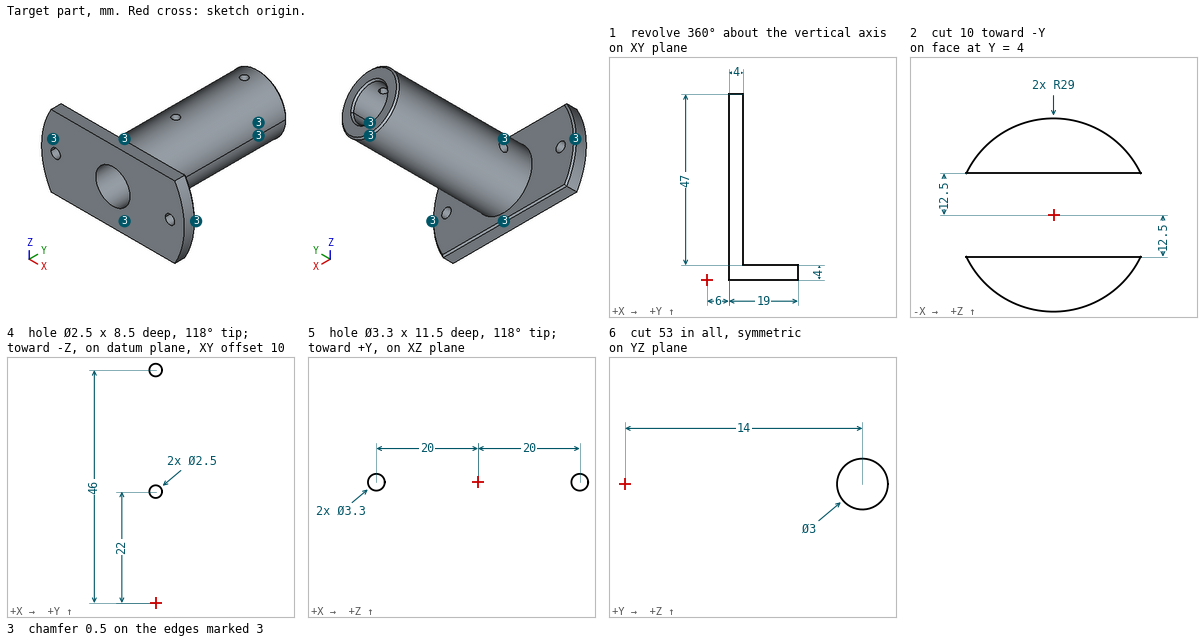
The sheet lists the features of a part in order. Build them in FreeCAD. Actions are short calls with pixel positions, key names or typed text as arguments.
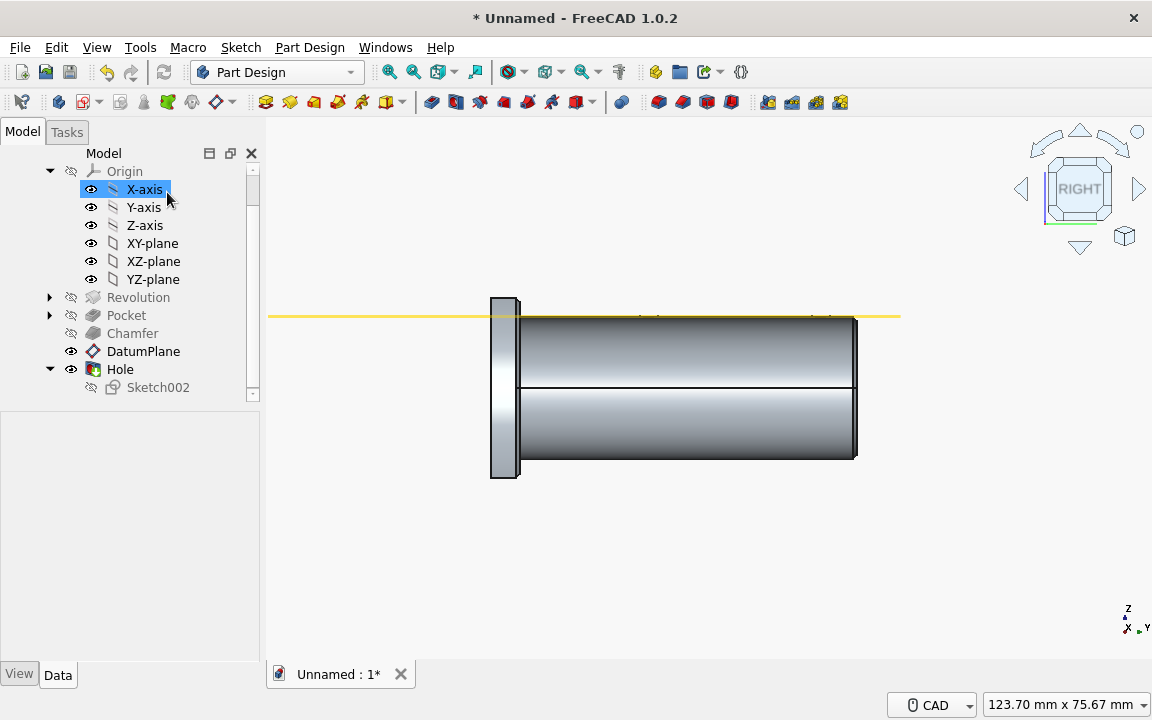
click(116, 351)
key(space)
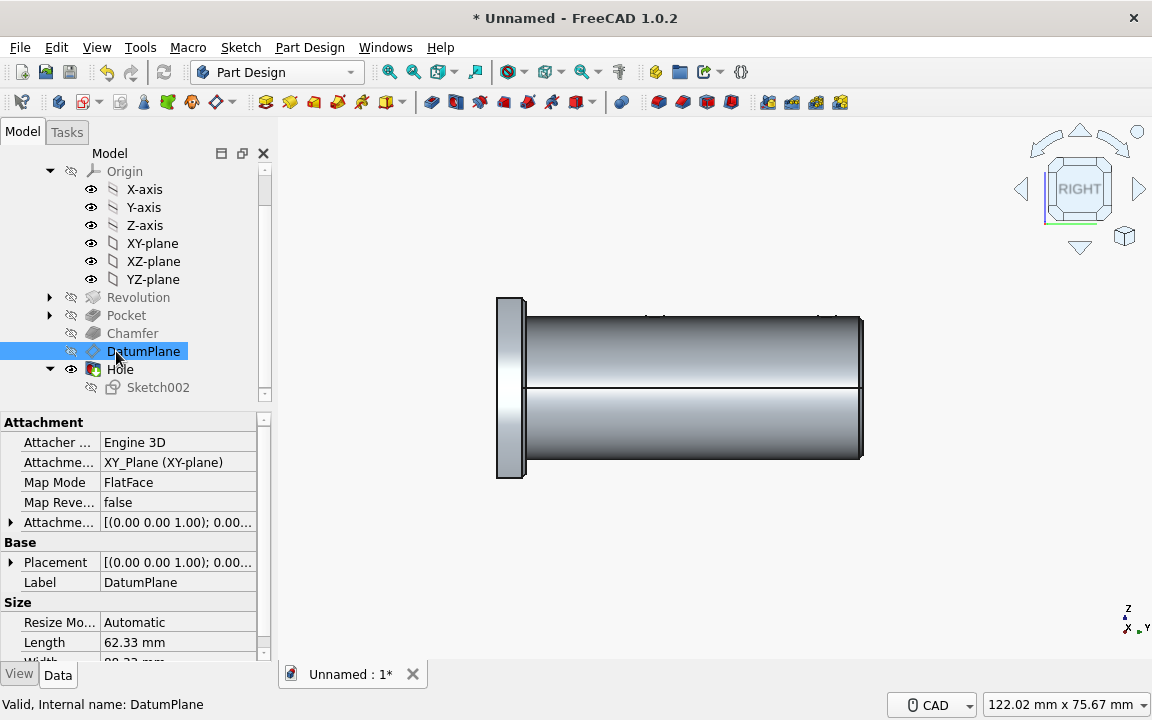
click(390, 72)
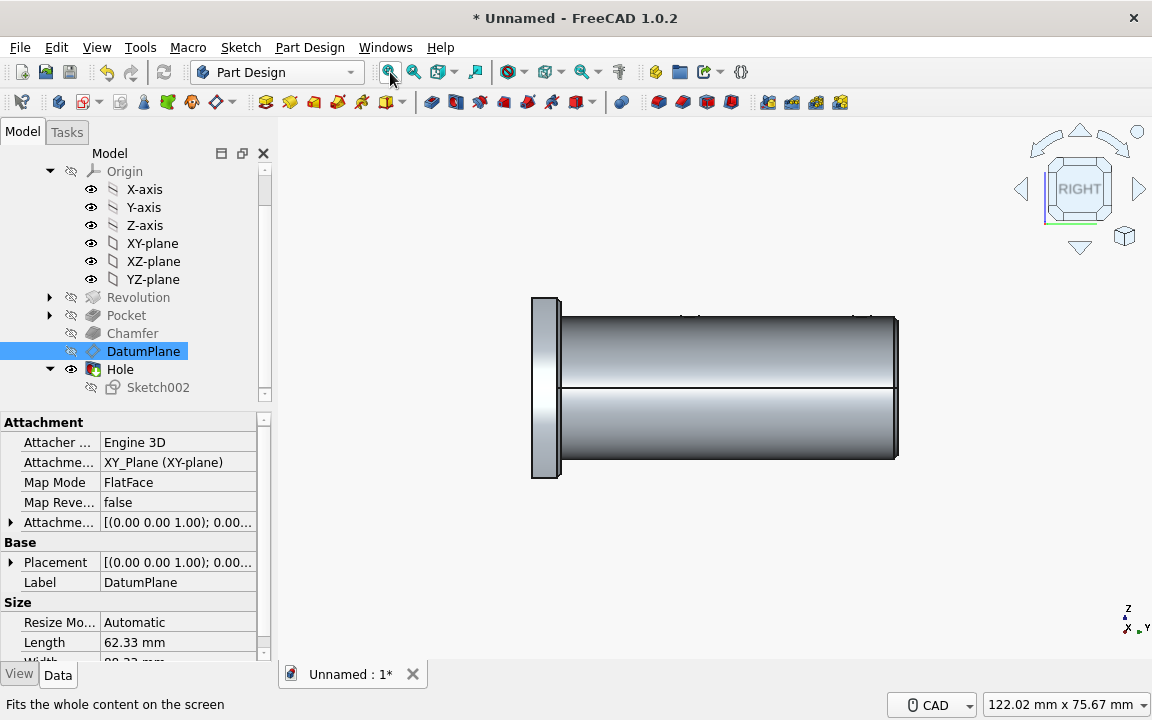
click(318, 619)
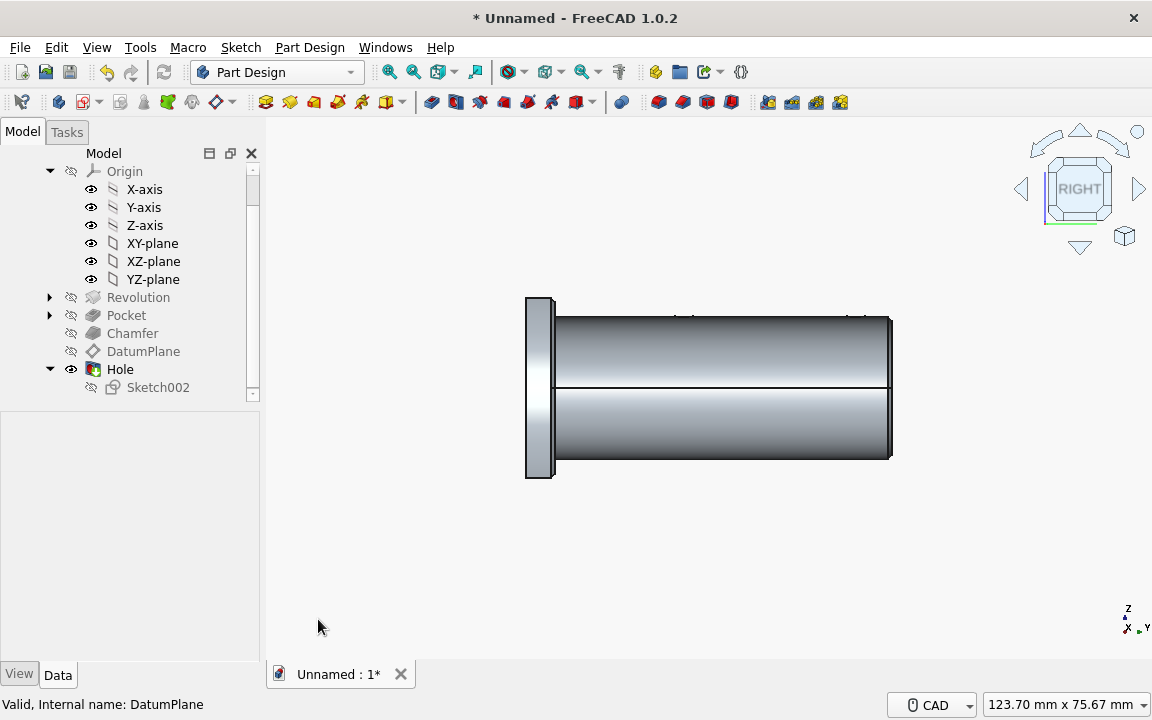
click(84, 102)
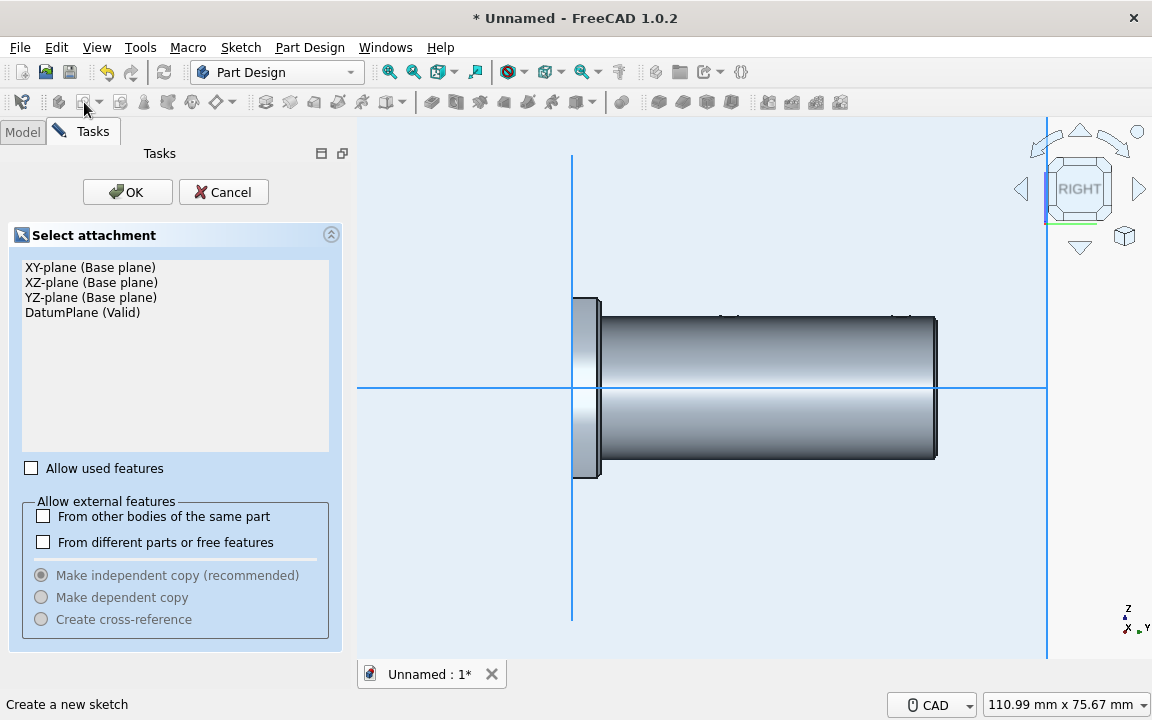
click(82, 282)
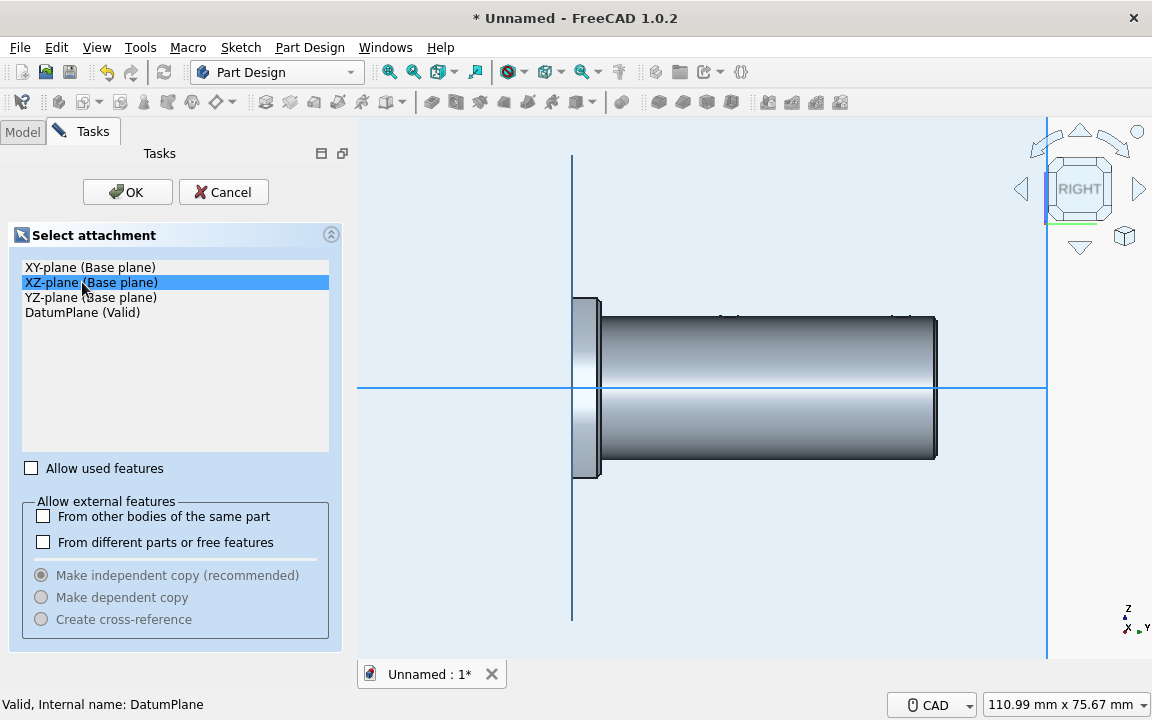
click(128, 192)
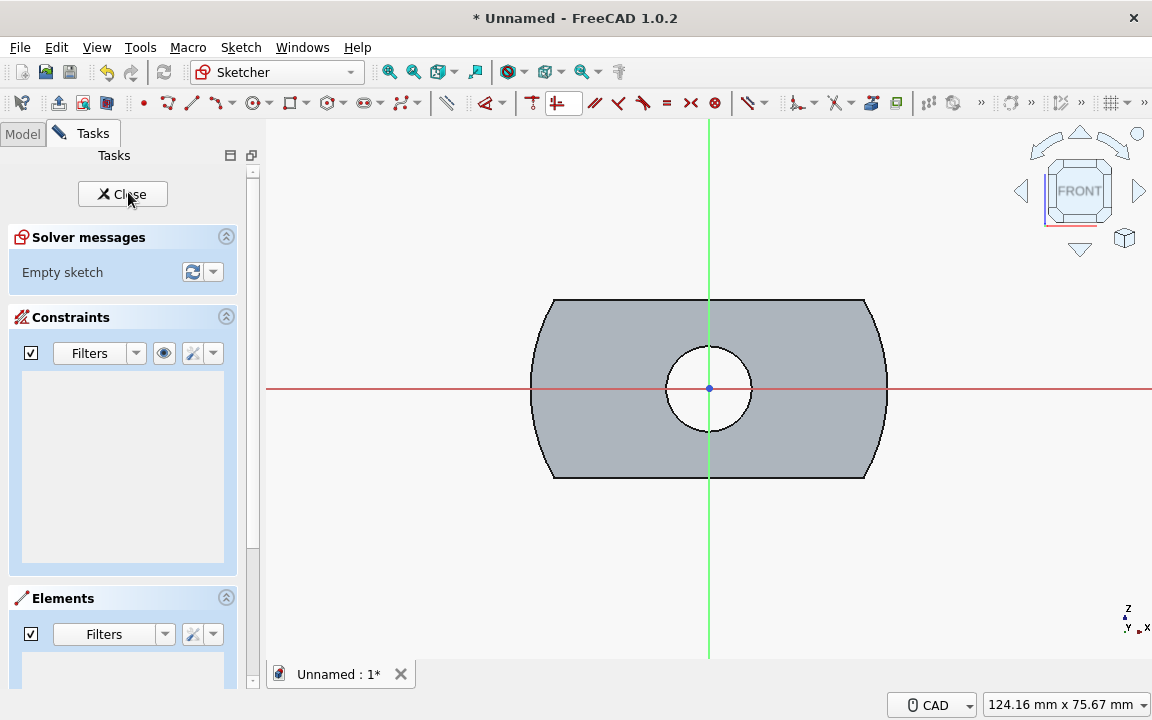
scroll(848, 389, up, 2)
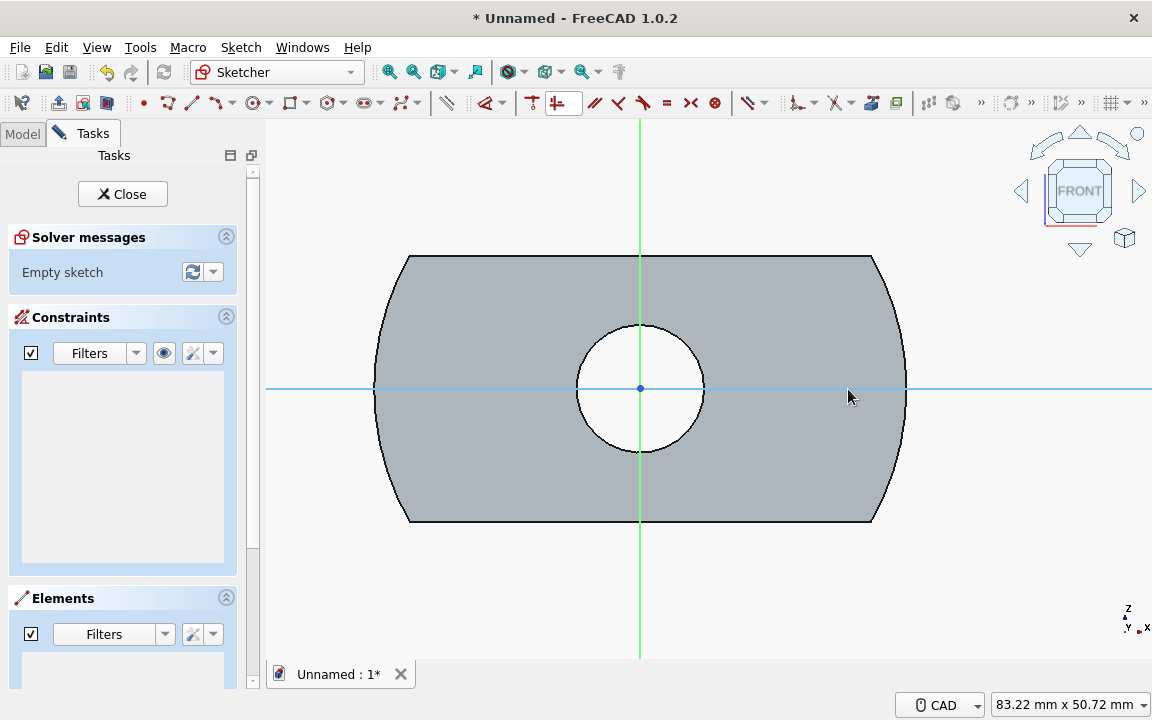
click(254, 104)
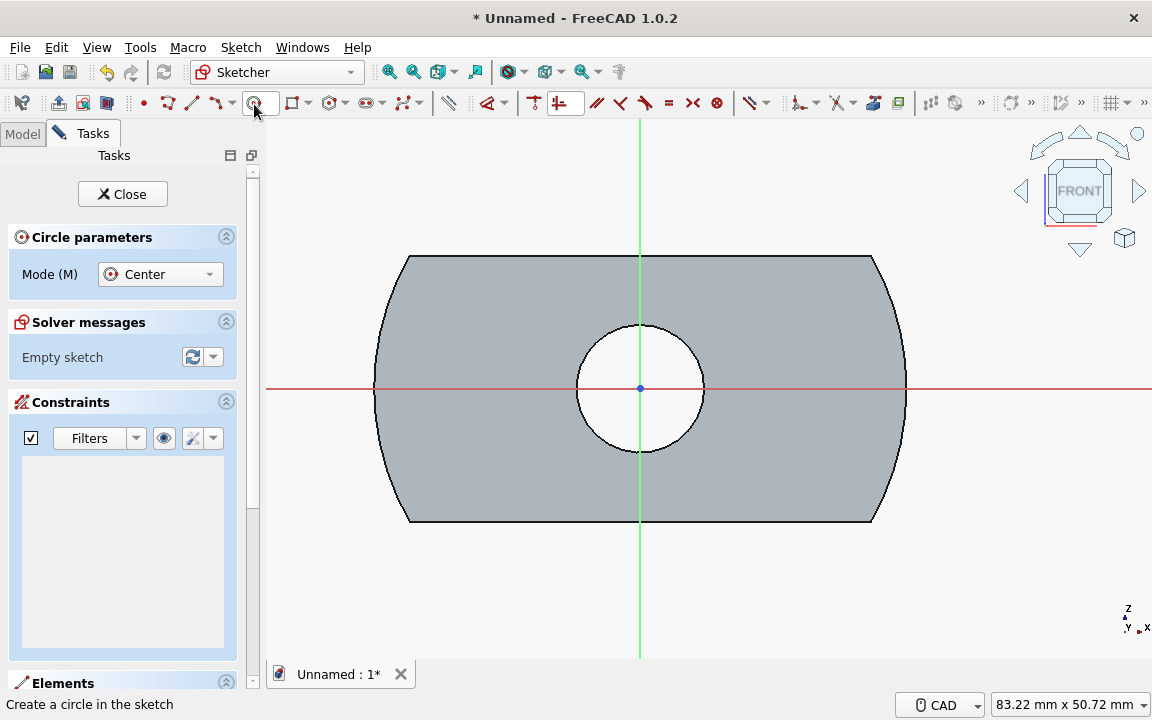
scroll(427, 389, up, 2)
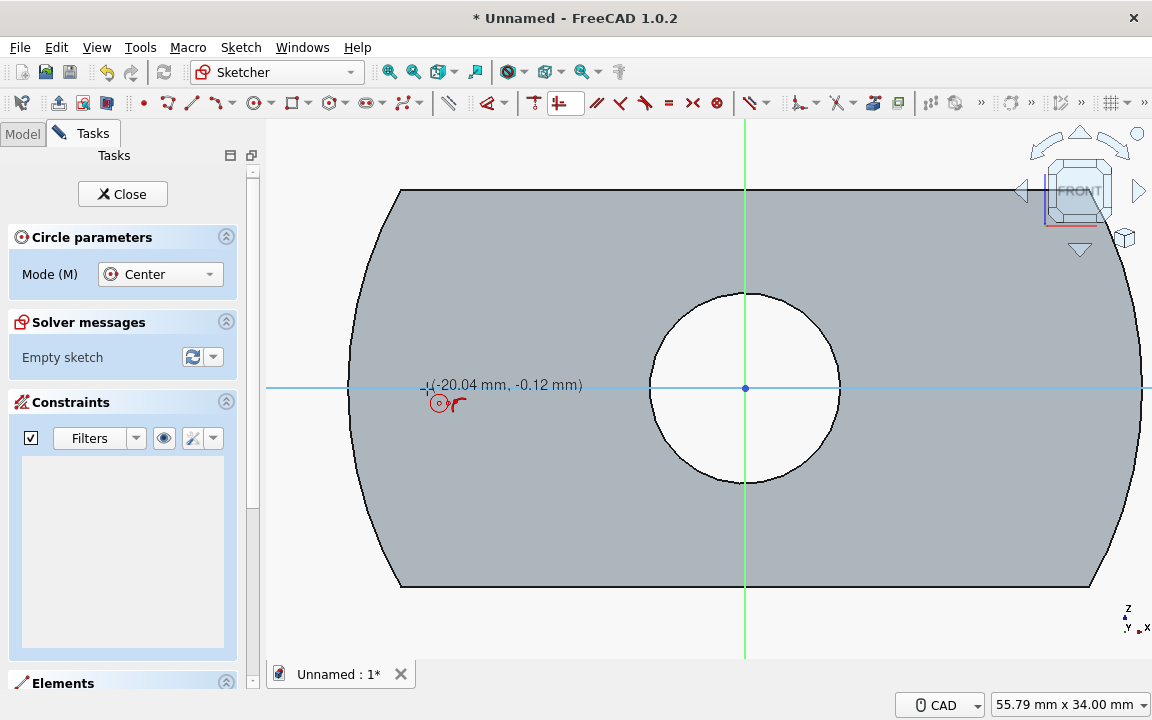
click(427, 388)
move(446, 370)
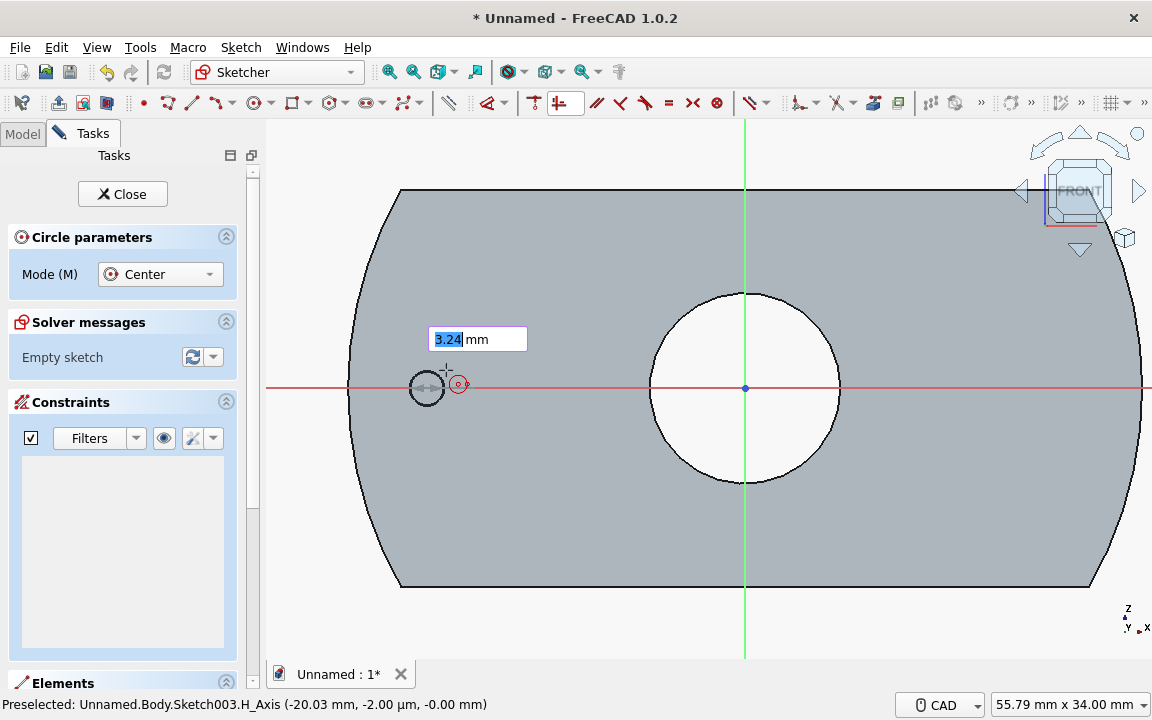
text(3.3)
key(Return)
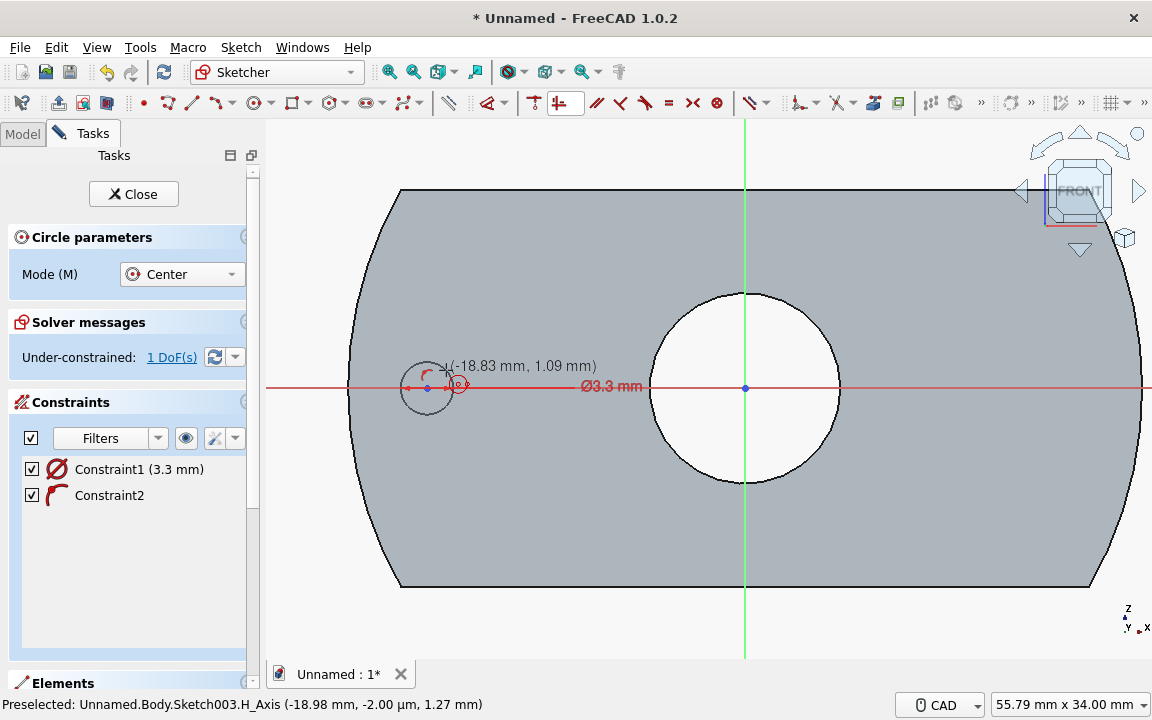
scroll(428, 390, down, 2)